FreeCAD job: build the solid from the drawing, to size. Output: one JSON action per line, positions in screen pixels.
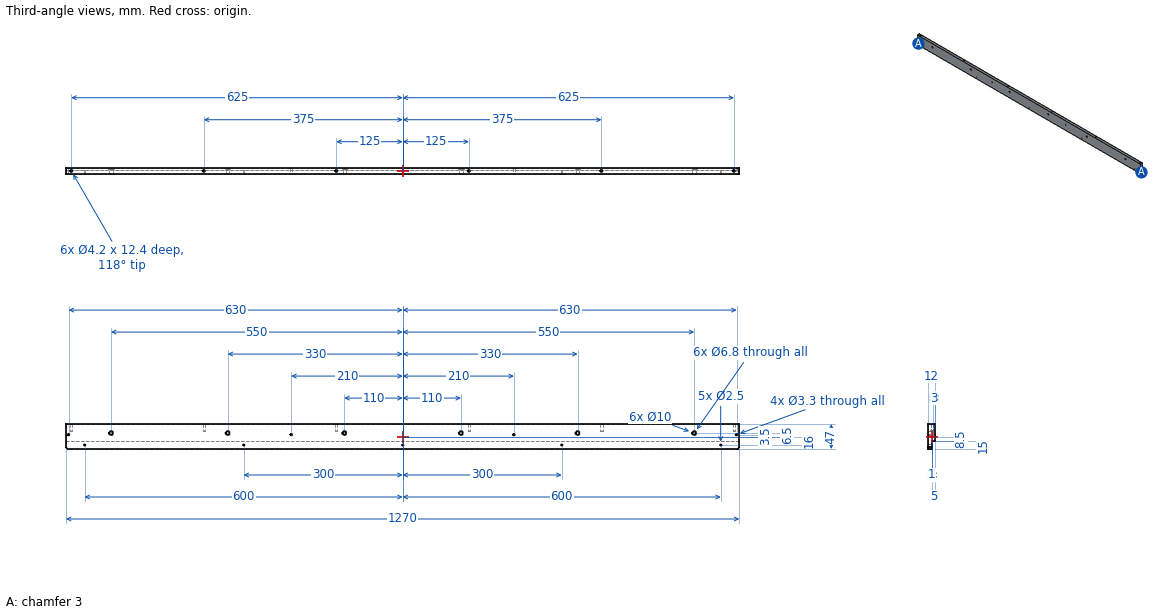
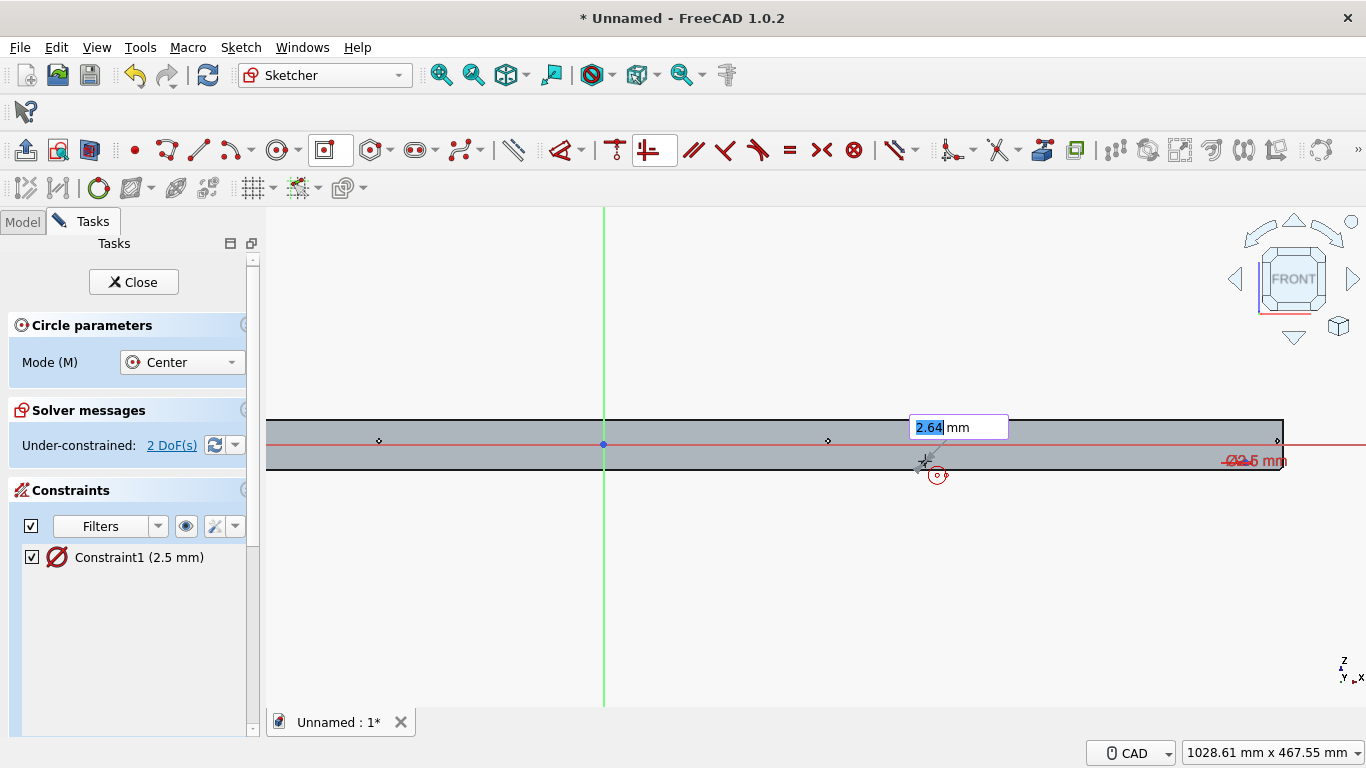
{"action": "type", "text": "2.5"}
{"action": "key", "text": "Return"}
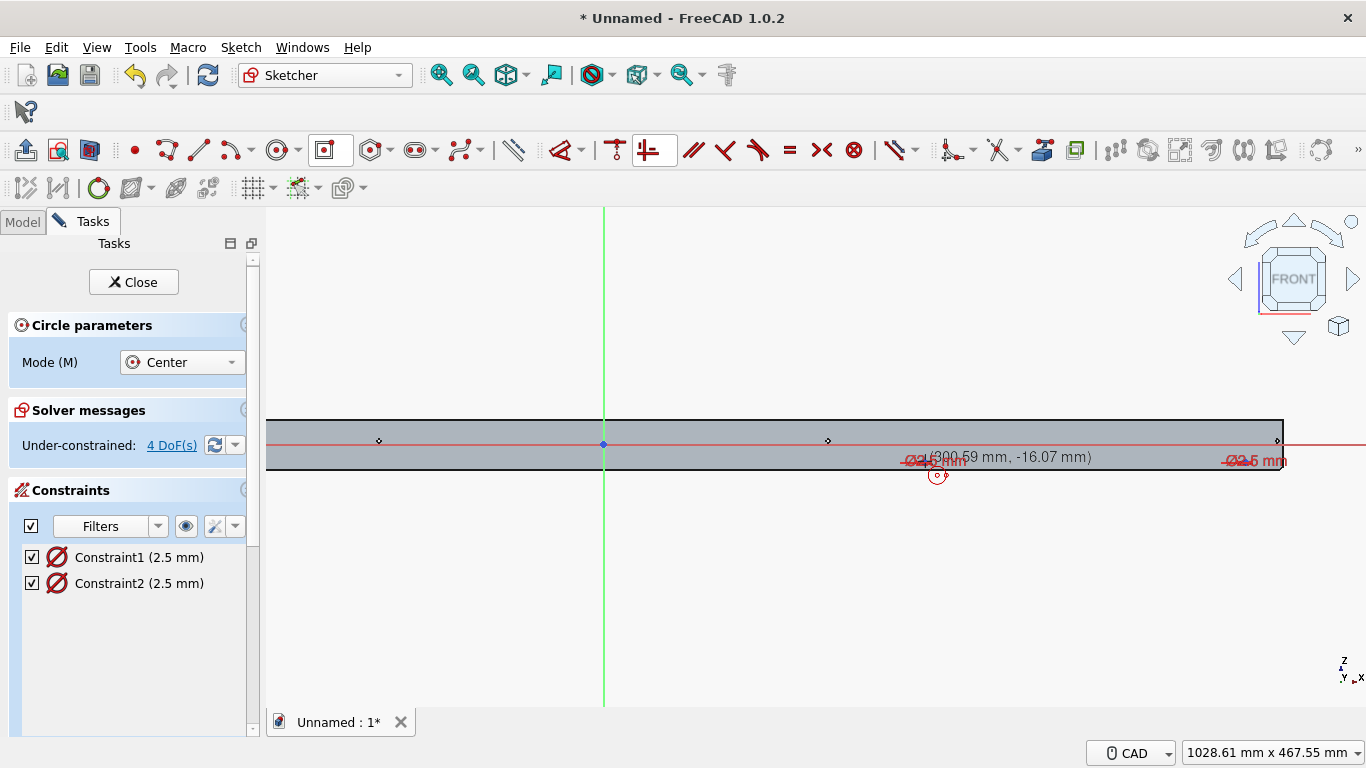
{"action": "scroll", "coordinate": [604, 462], "scroll_direction": "up", "scroll_amount": 15}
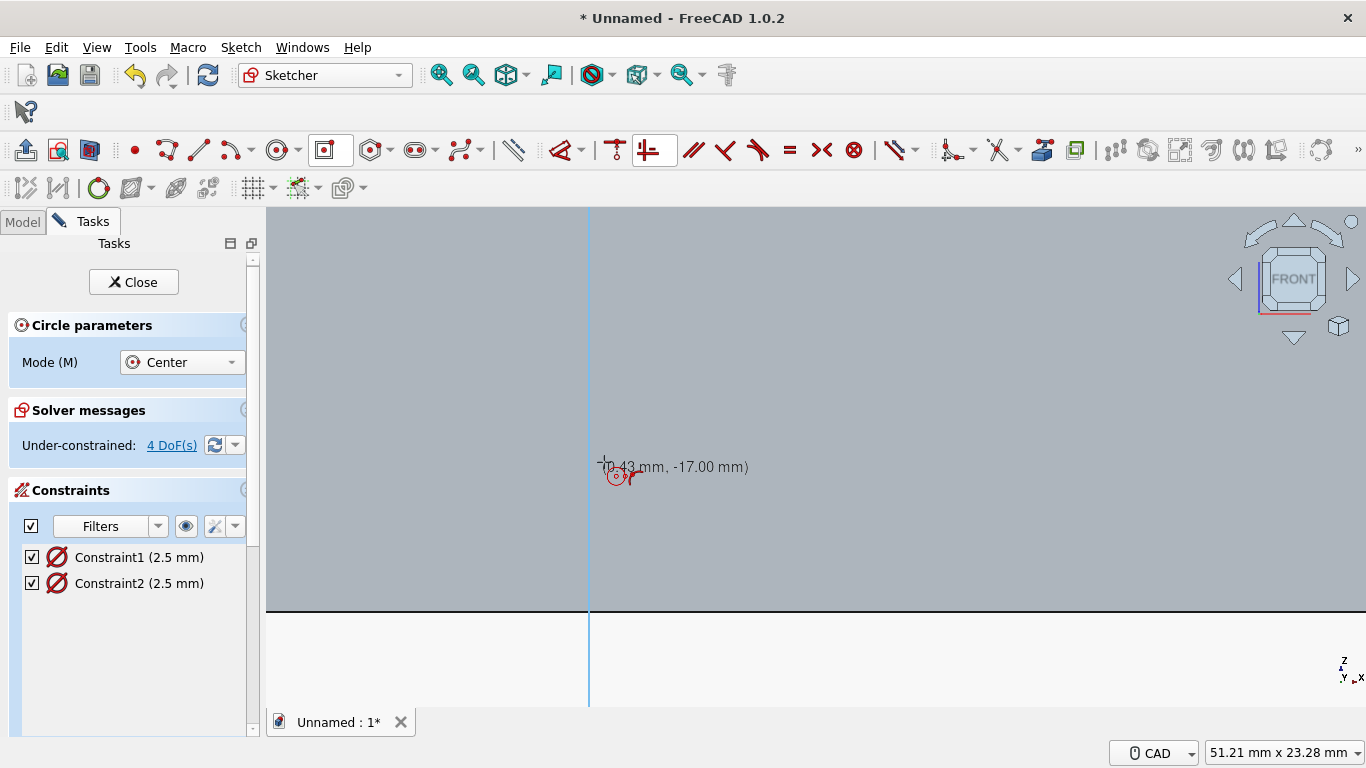
{"action": "scroll", "coordinate": [752, 462], "scroll_direction": "down", "scroll_amount": 18}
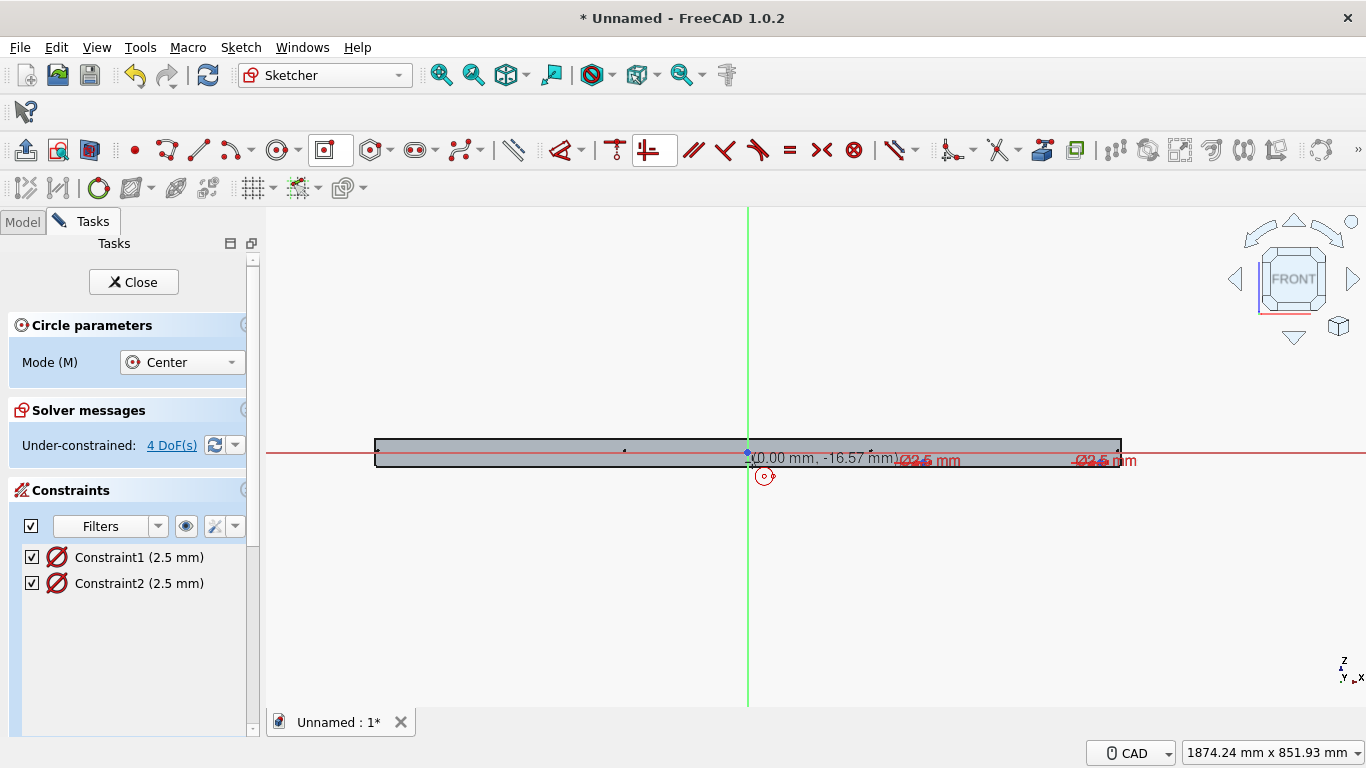
{"action": "scroll", "coordinate": [748, 462], "scroll_direction": "up", "scroll_amount": 3}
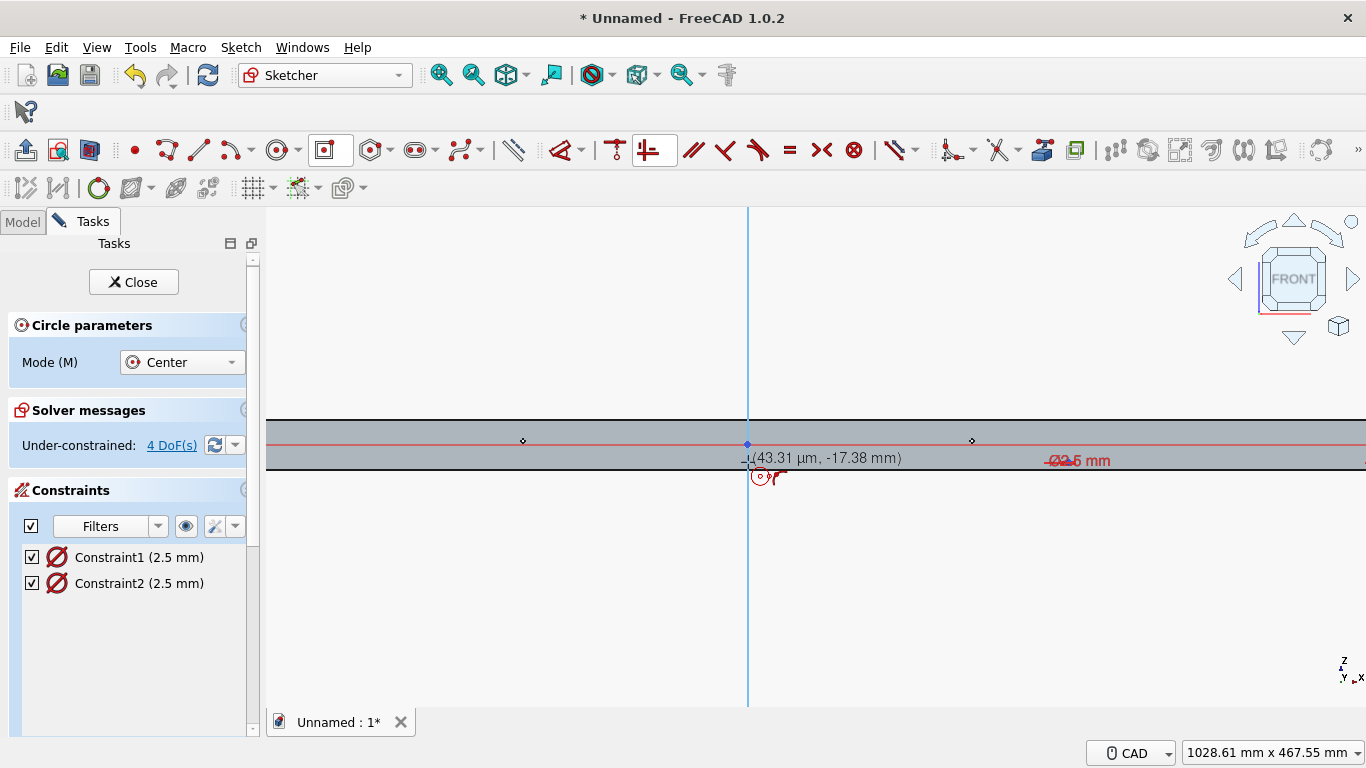
{"action": "left_click", "coordinate": [748, 462]}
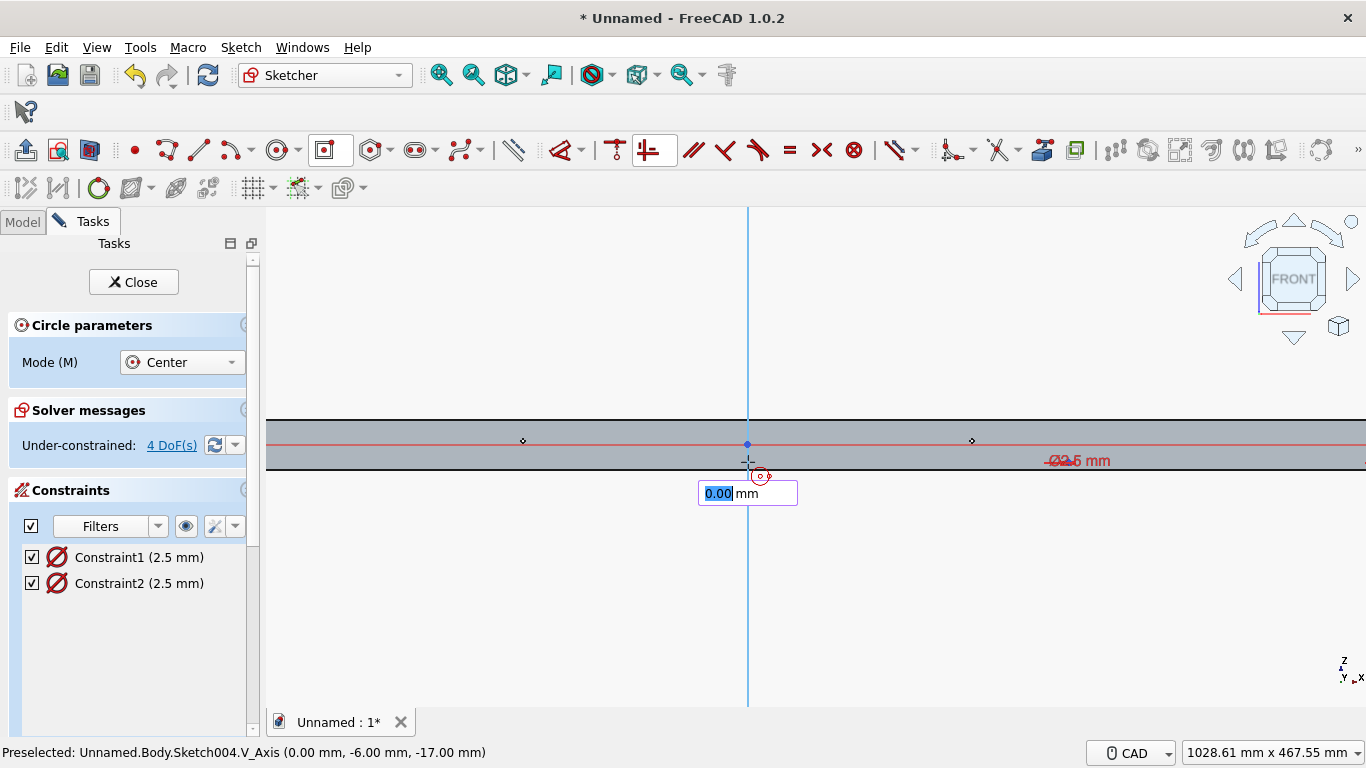
{"action": "scroll", "coordinate": [749, 461], "scroll_direction": "up", "scroll_amount": 13}
{"action": "mouse_move", "coordinate": [741, 461]}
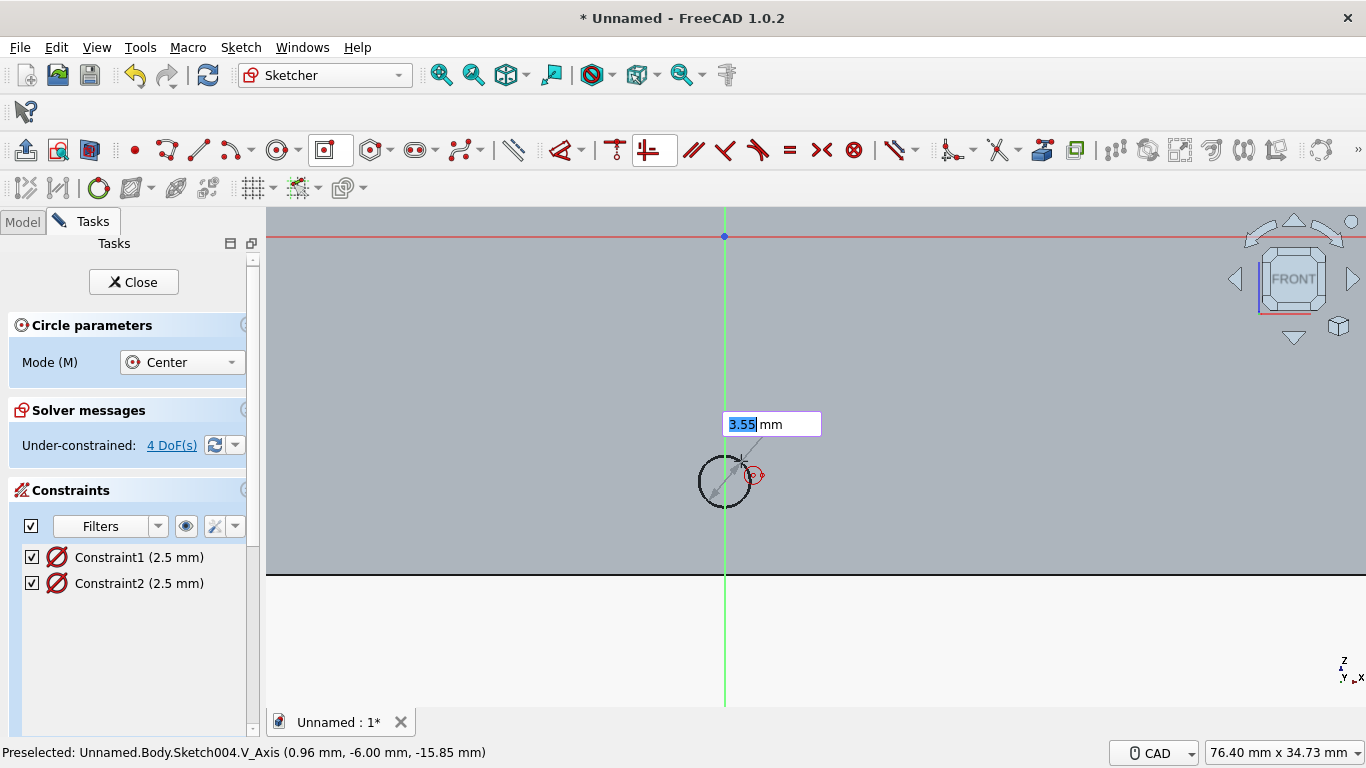
{"action": "type", "text": "2.5"}
{"action": "key", "text": "Return"}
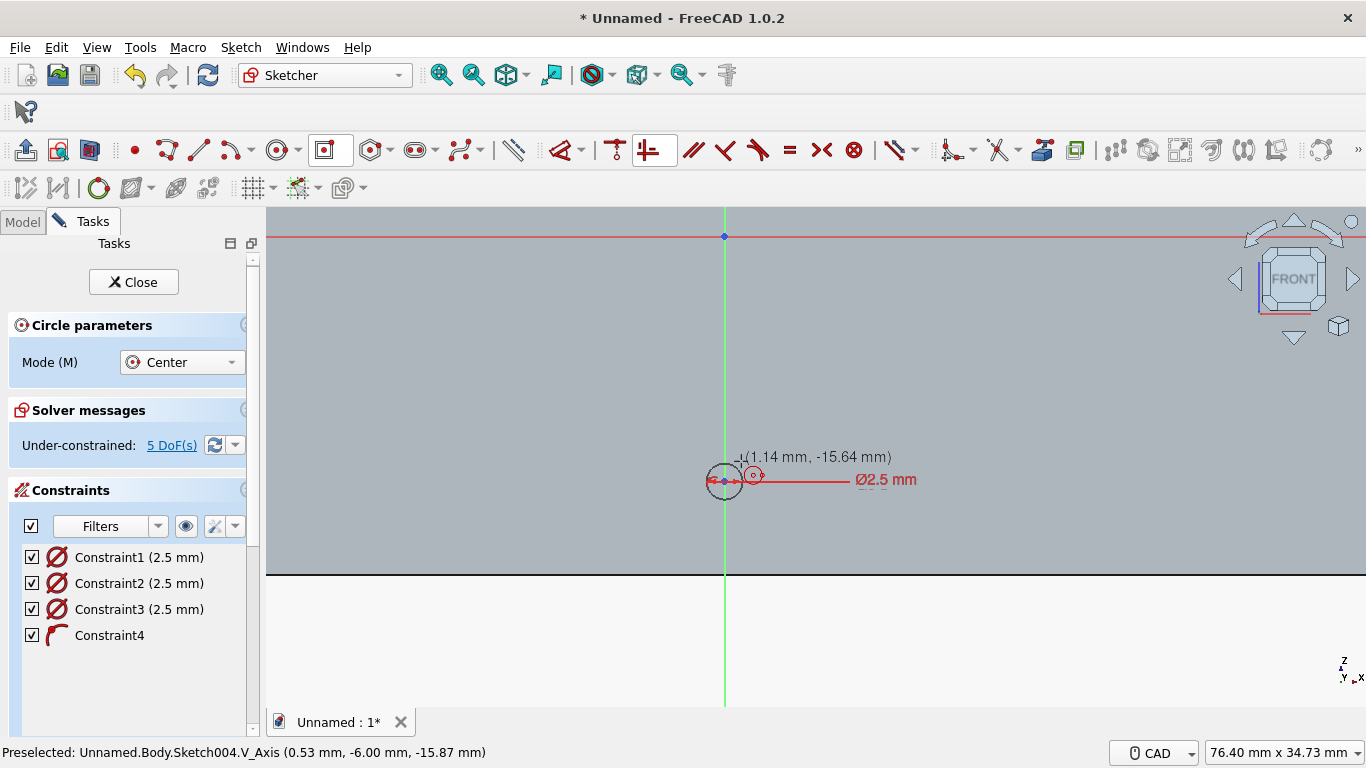
{"action": "scroll", "coordinate": [748, 461], "scroll_direction": "down", "scroll_amount": 16}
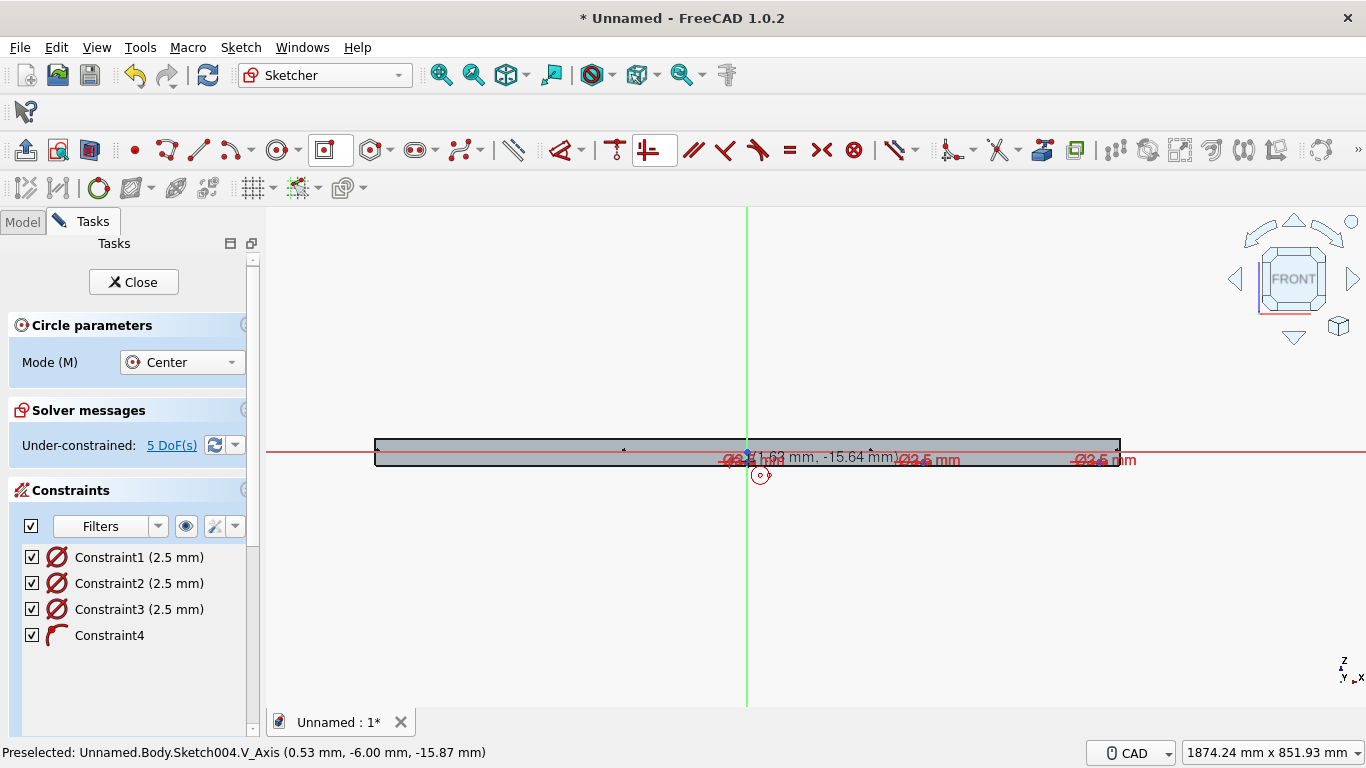
{"action": "scroll", "coordinate": [571, 462], "scroll_direction": "up", "scroll_amount": 18}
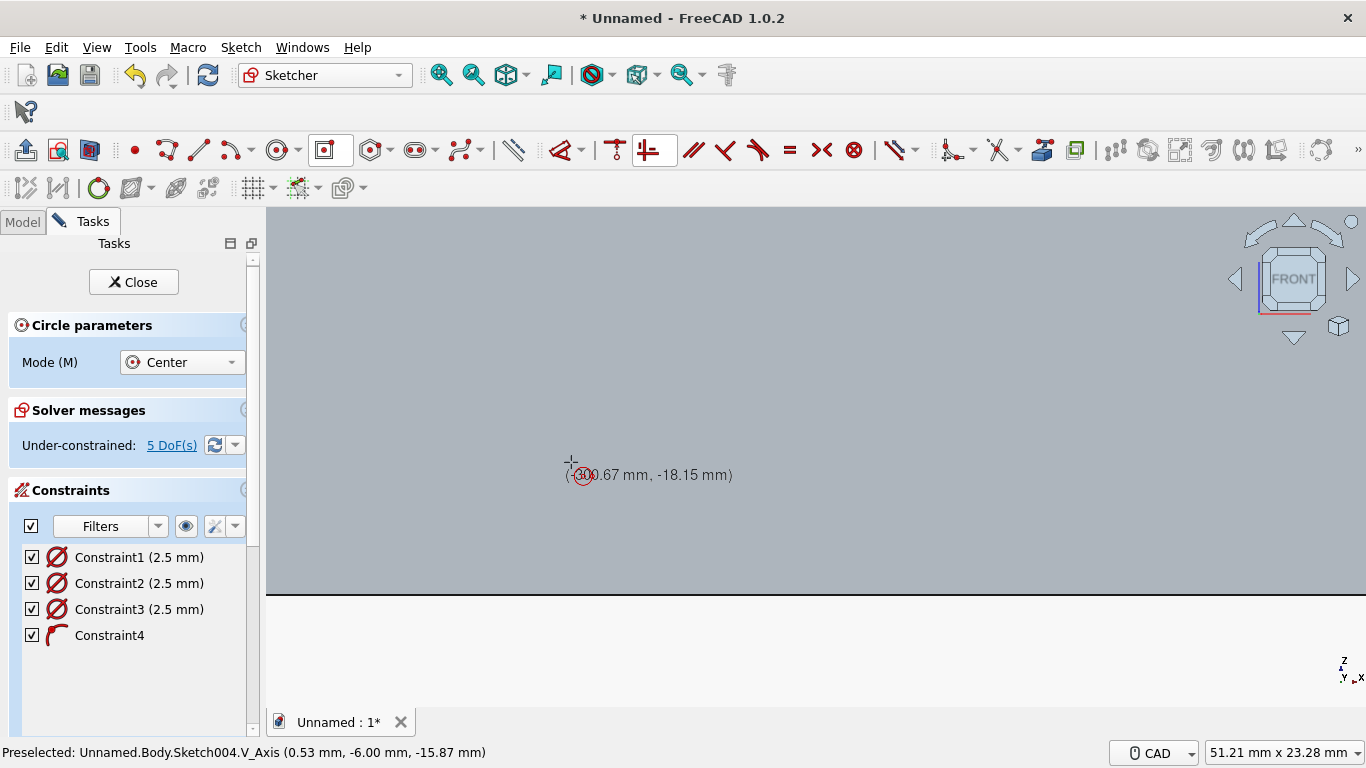
{"action": "scroll", "coordinate": [571, 462], "scroll_direction": "down", "scroll_amount": 18}